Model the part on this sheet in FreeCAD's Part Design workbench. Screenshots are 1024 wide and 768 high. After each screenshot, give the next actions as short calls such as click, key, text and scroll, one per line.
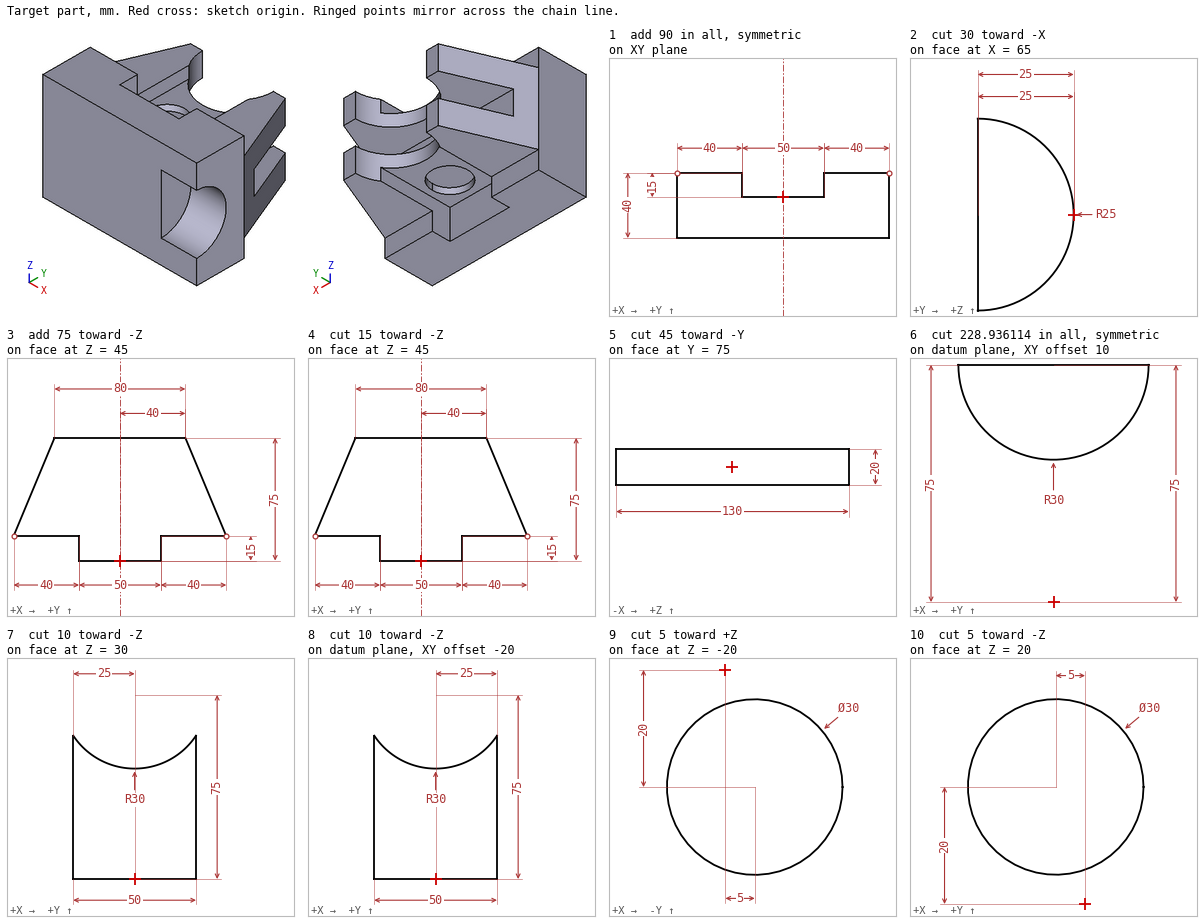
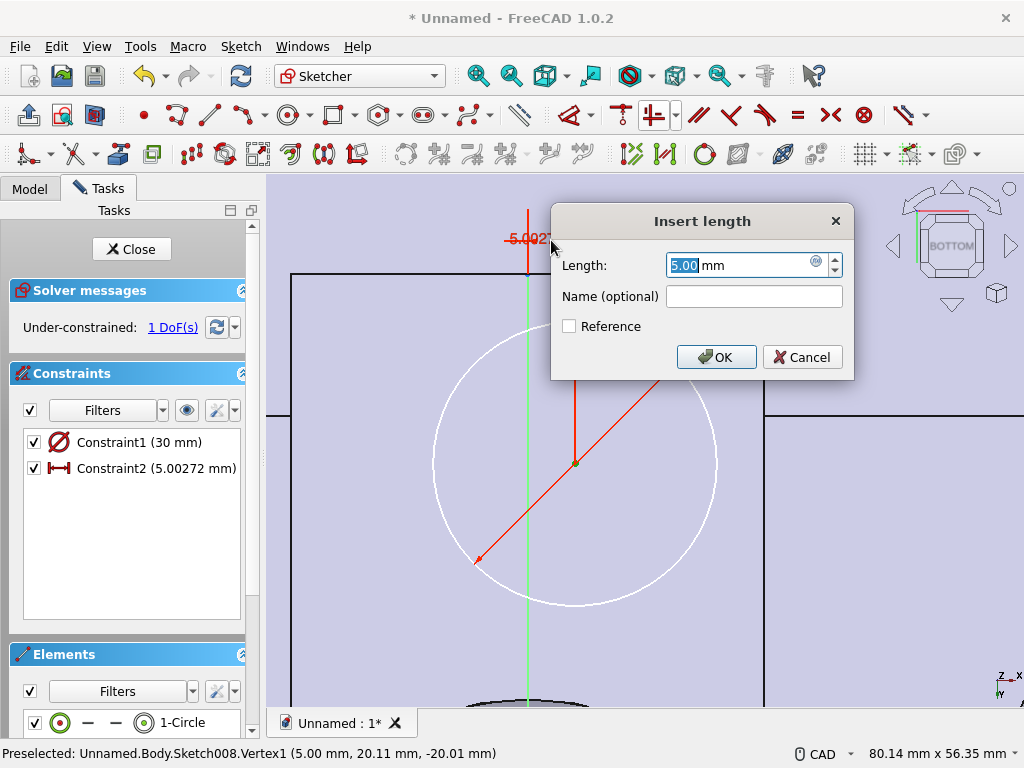
text(5)
key(Return)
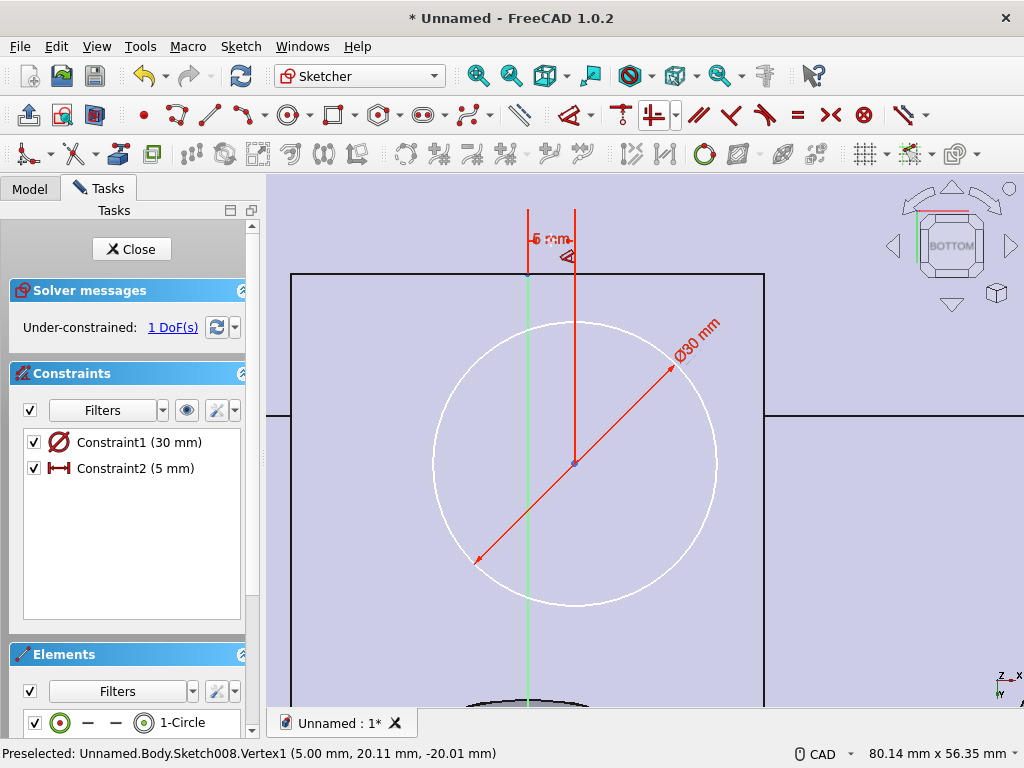
click(575, 464)
click(494, 369)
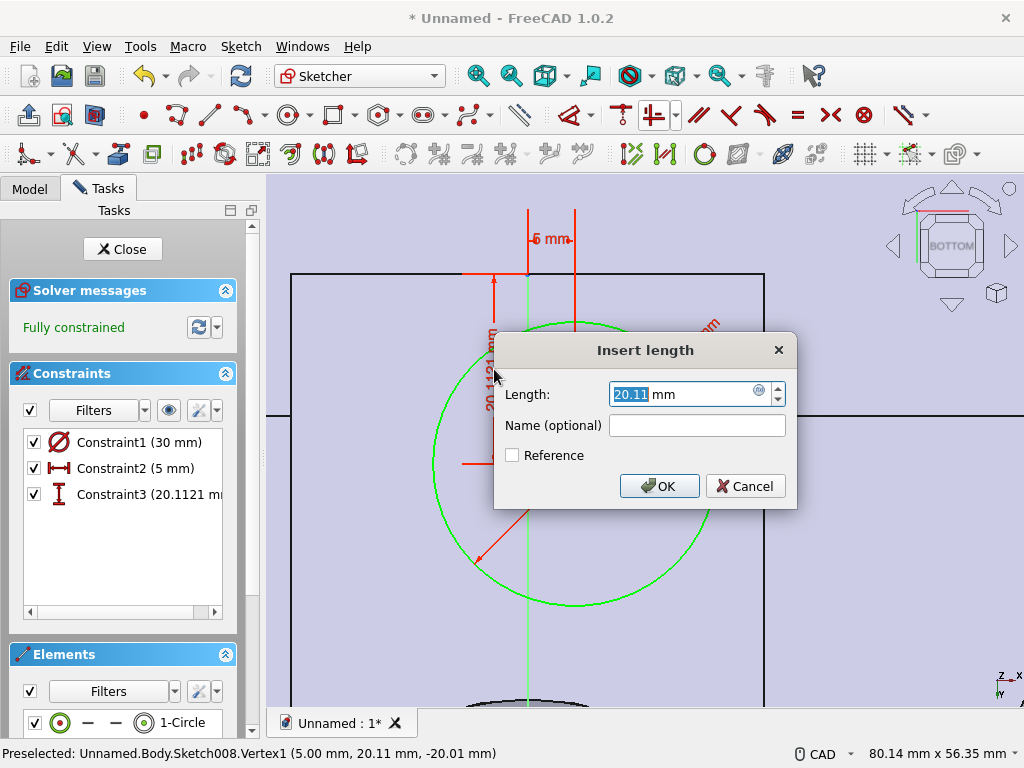
text(20)
key(Return)
key(Escape)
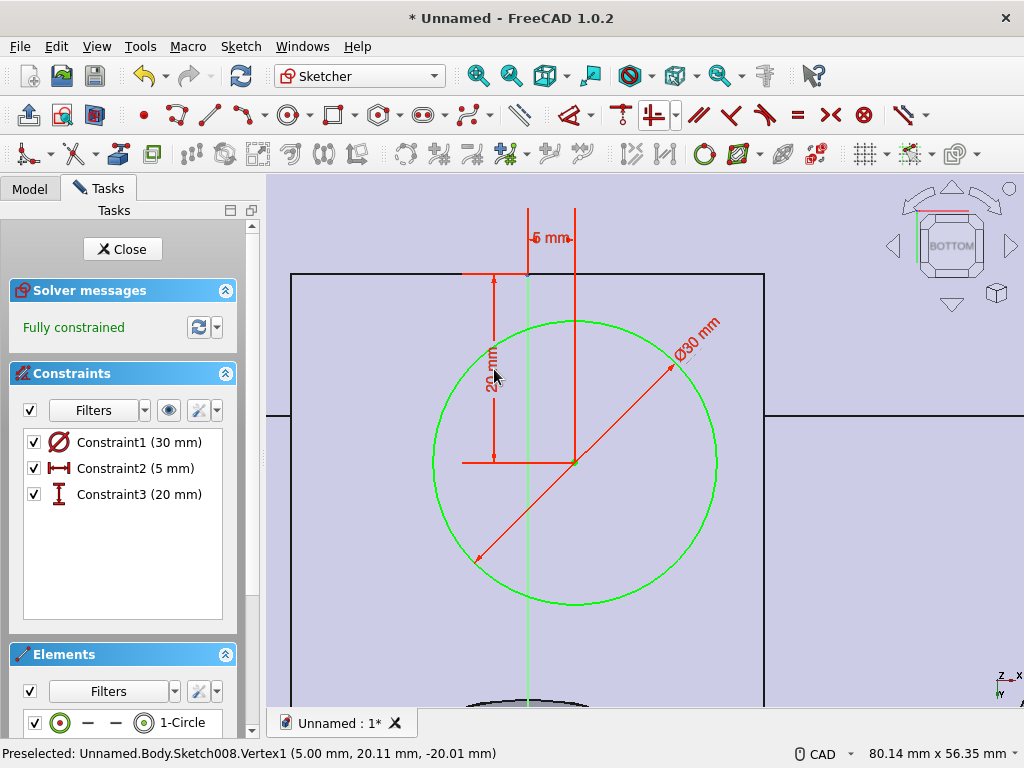
click(123, 249)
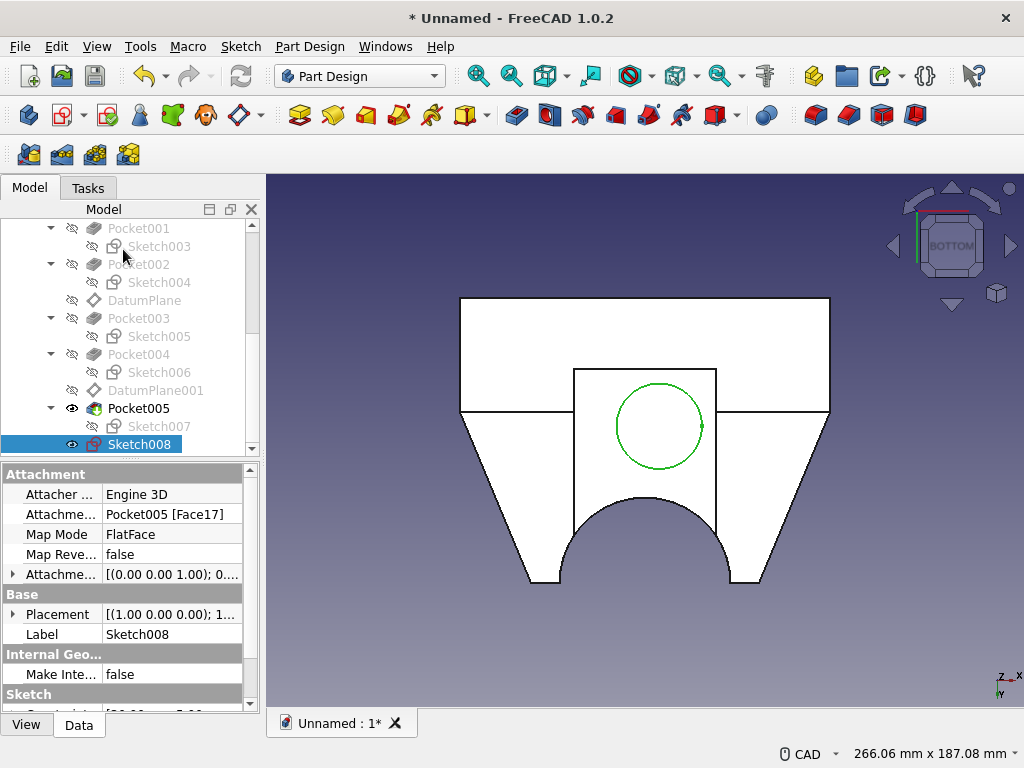
click(517, 116)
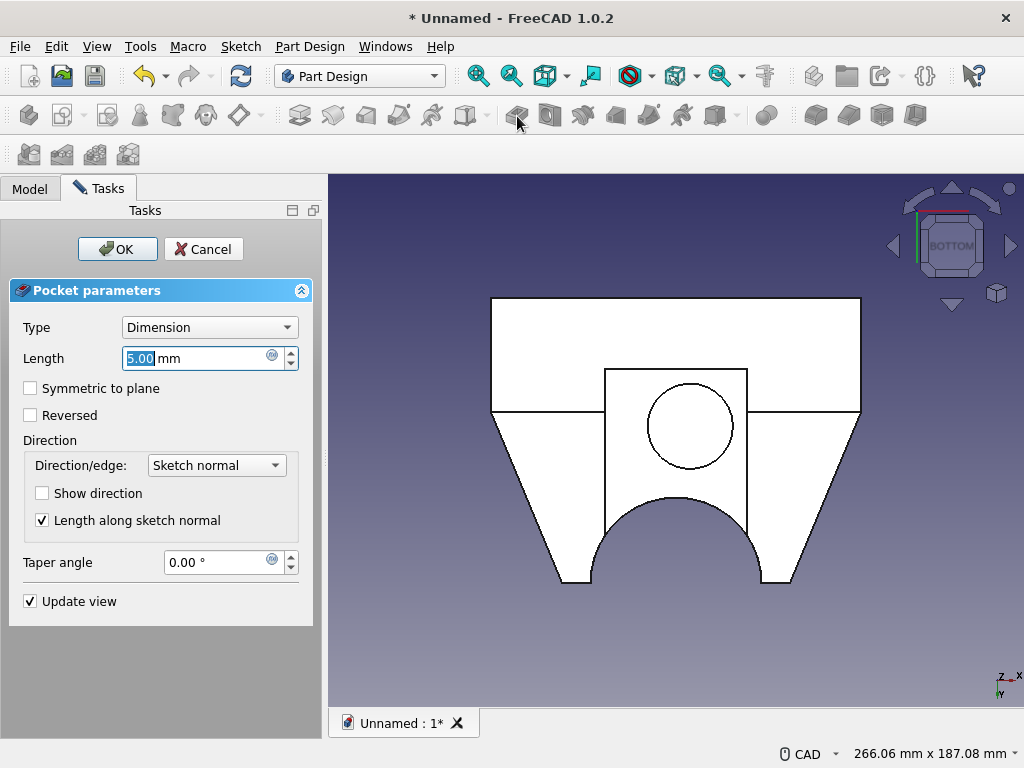
text(5)
key(Tab)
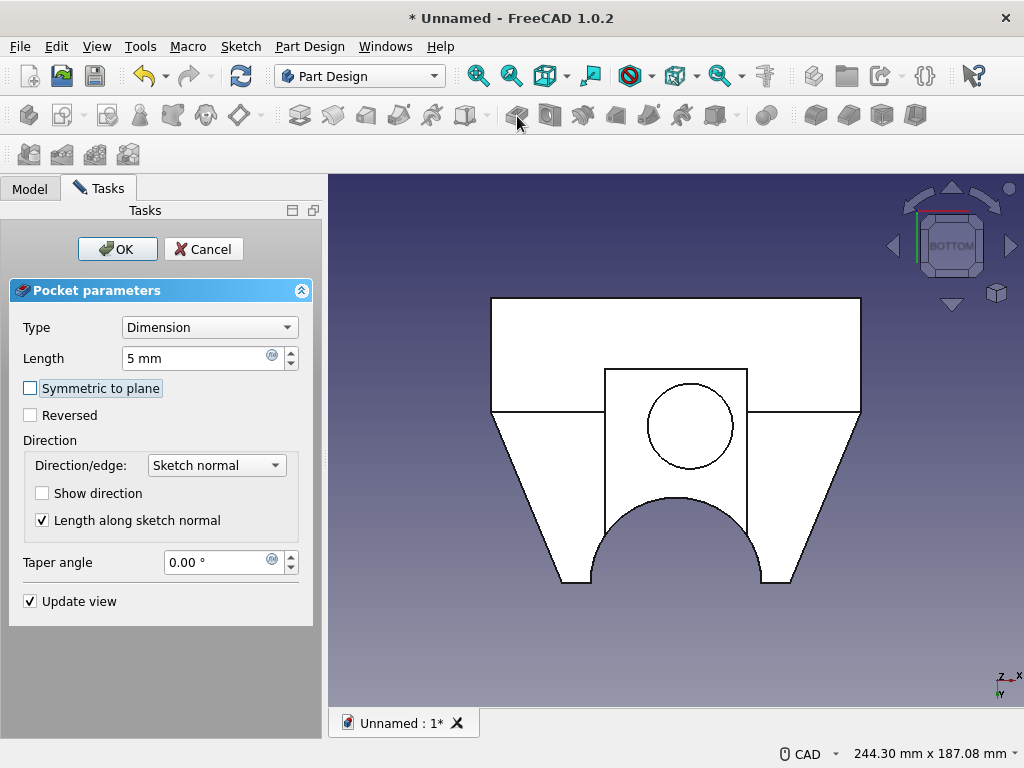
click(118, 249)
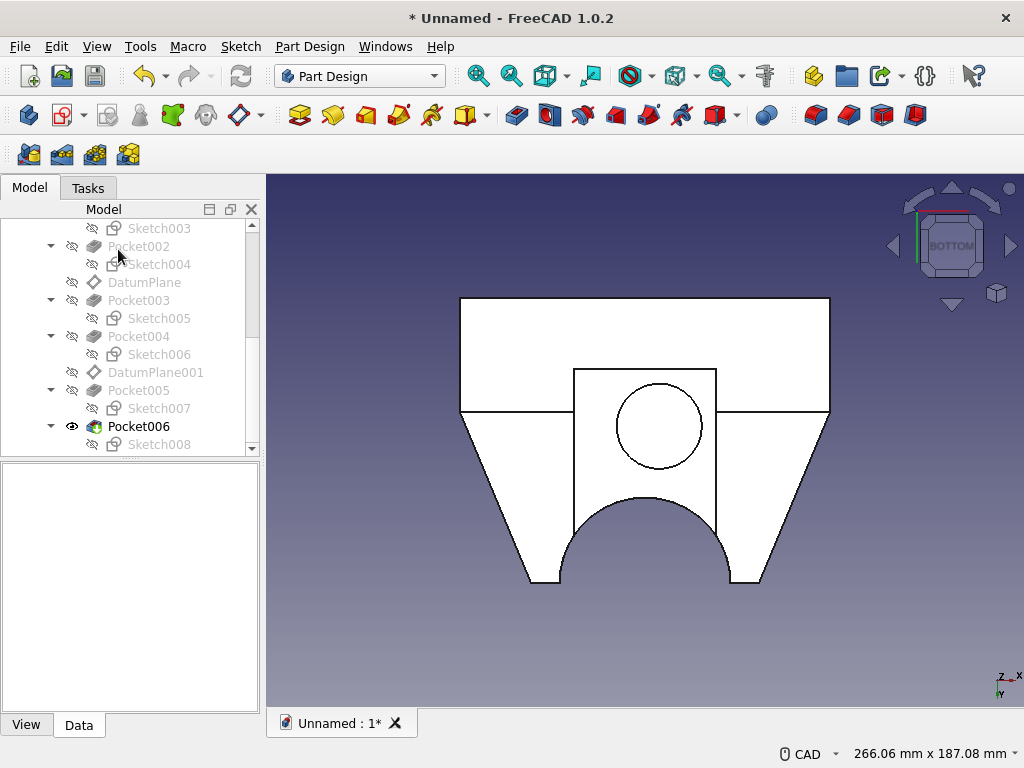
key(0)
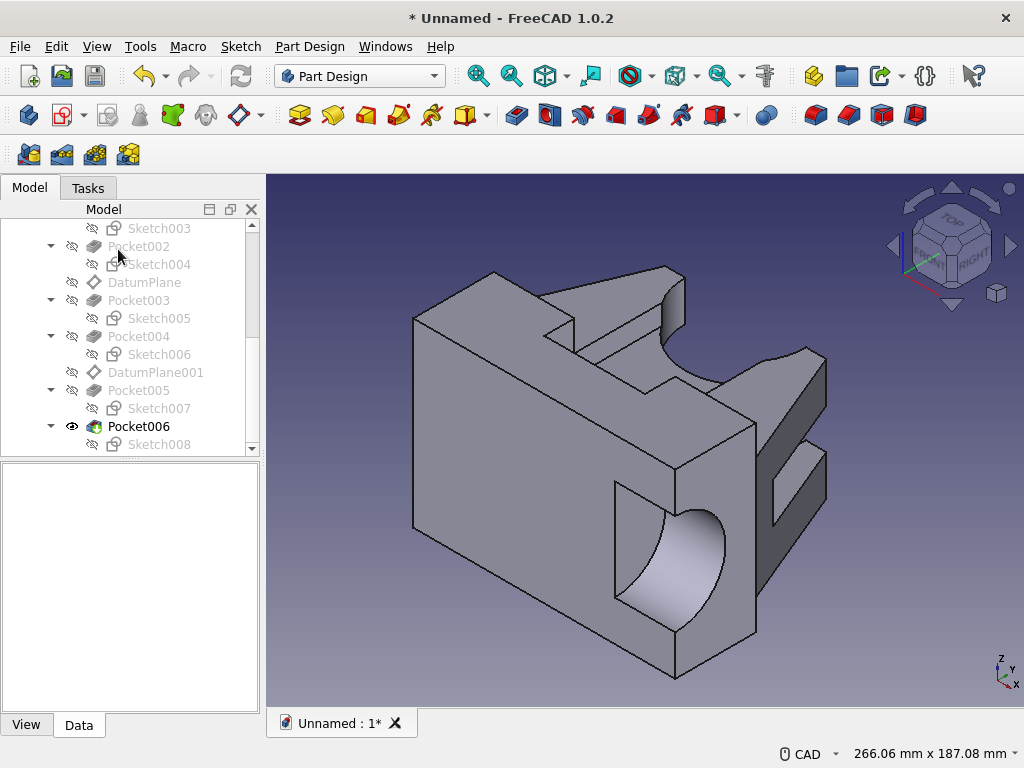
key(2)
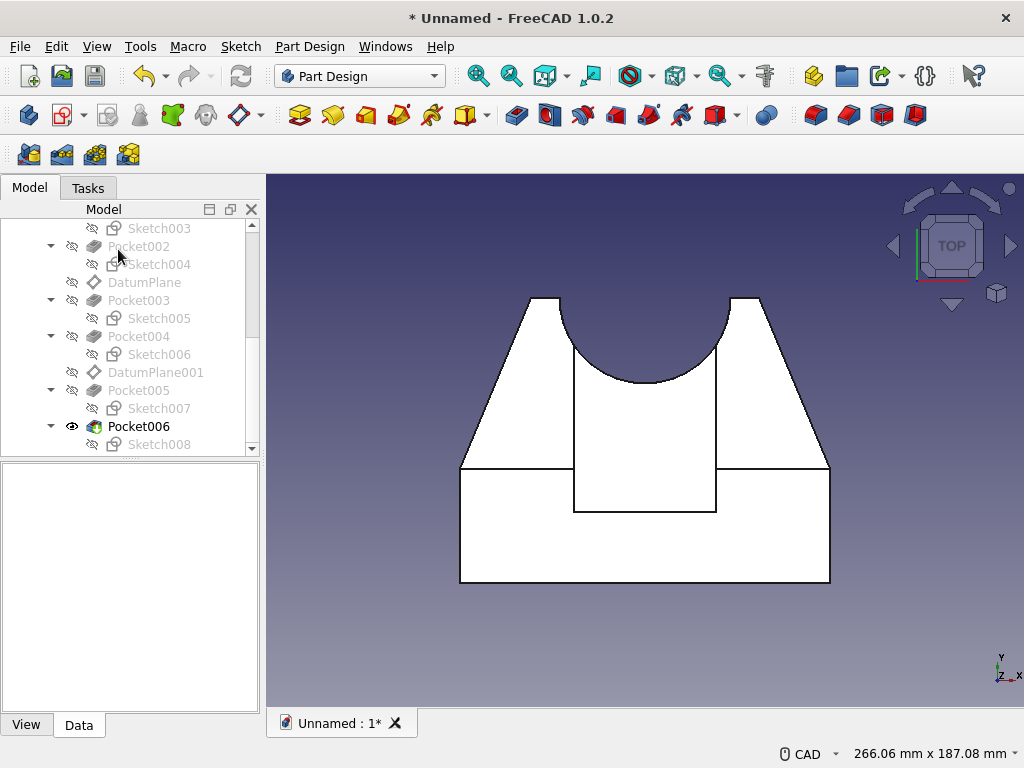
click(645, 451)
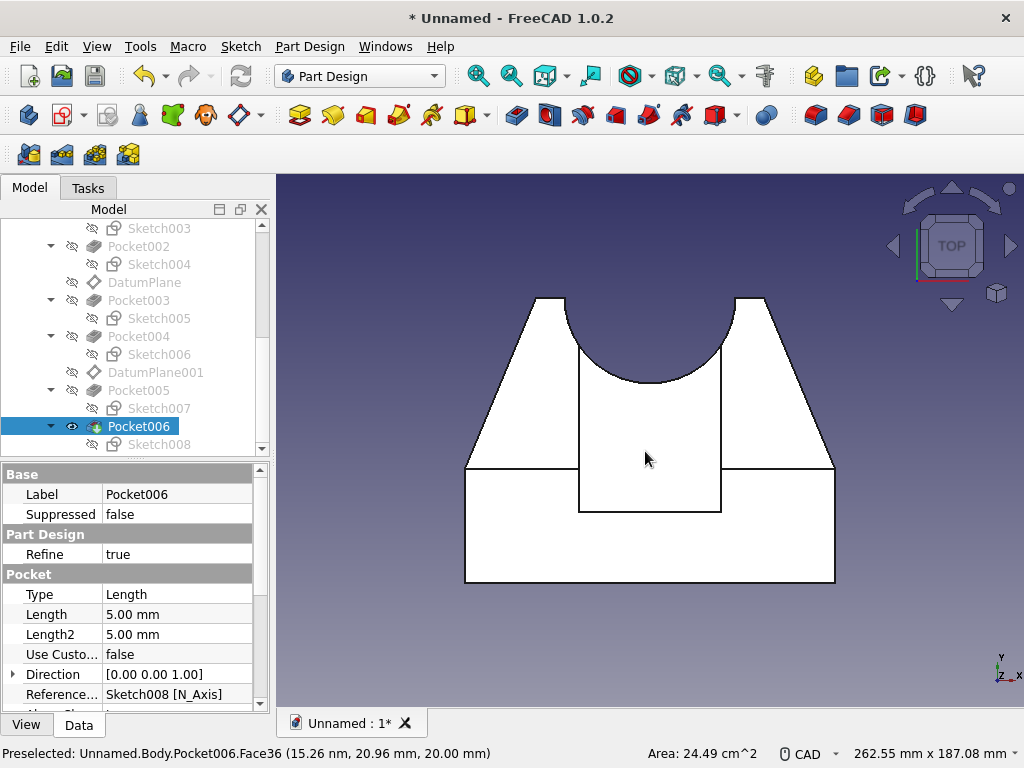
click(62, 116)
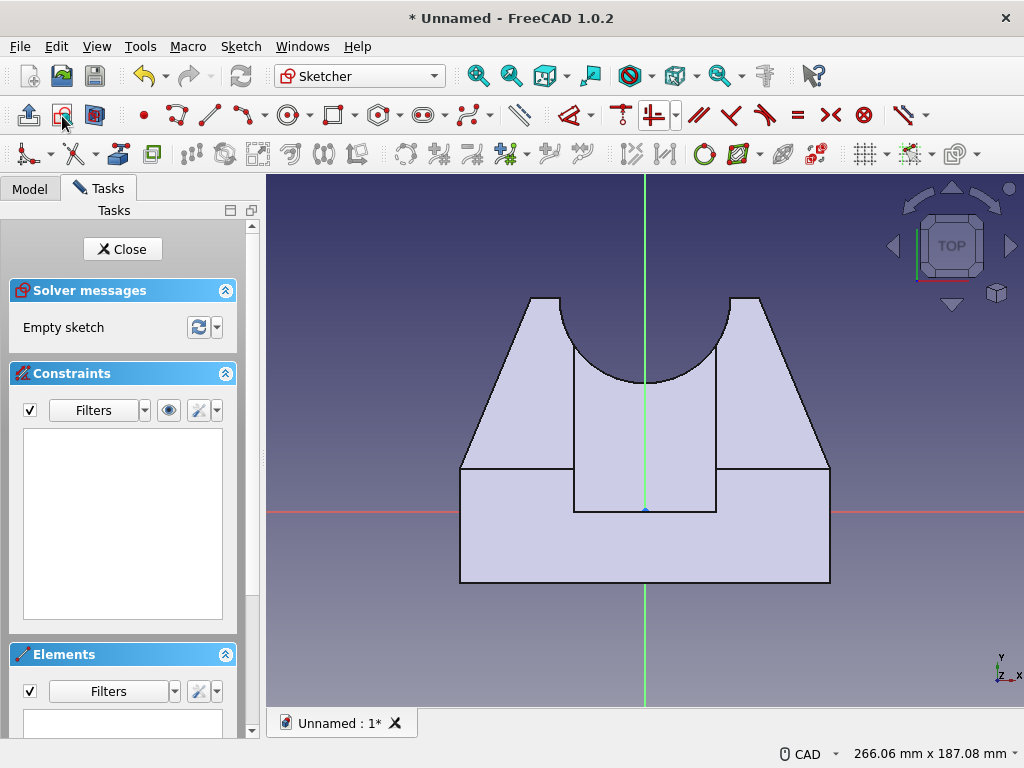
key(q)
key(s)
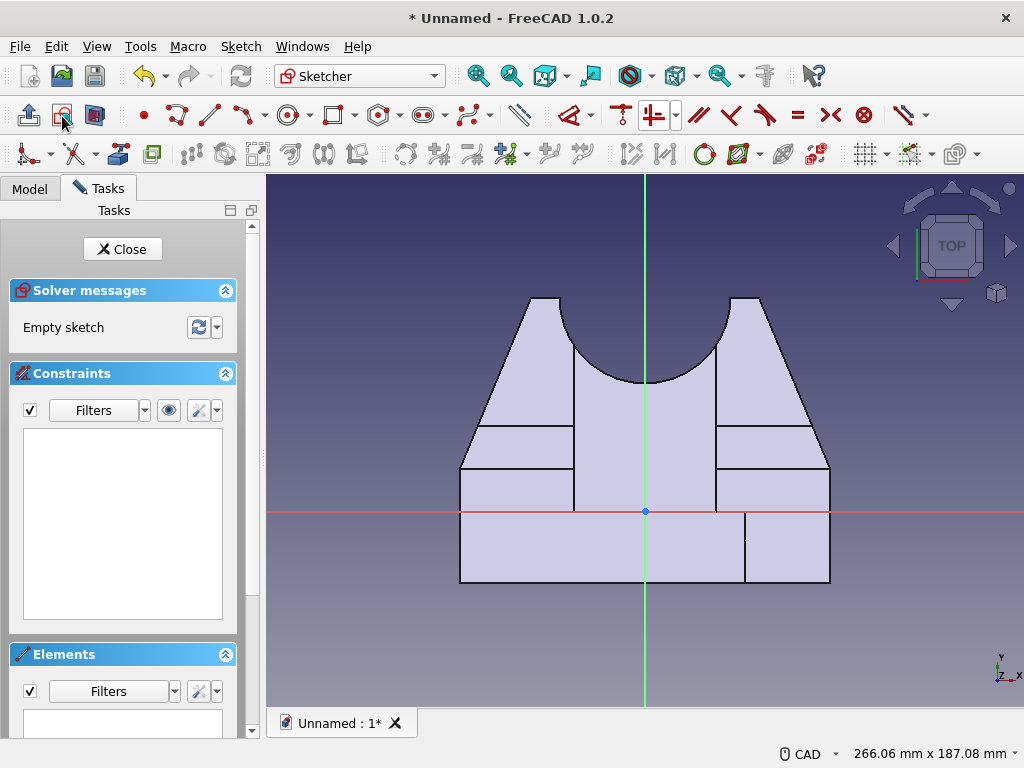
scroll(654, 471, up, 6)